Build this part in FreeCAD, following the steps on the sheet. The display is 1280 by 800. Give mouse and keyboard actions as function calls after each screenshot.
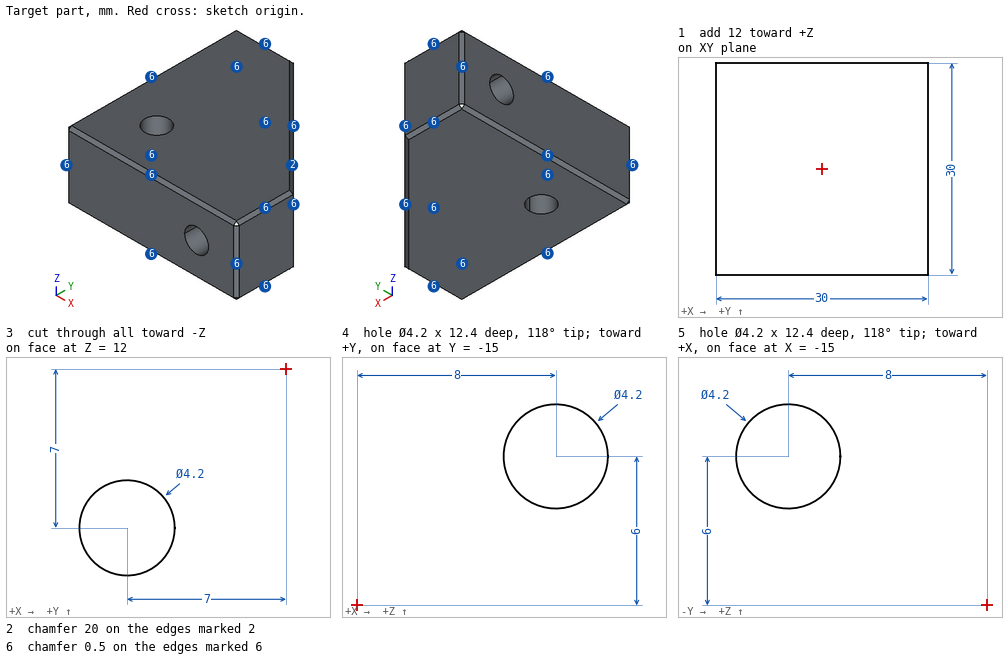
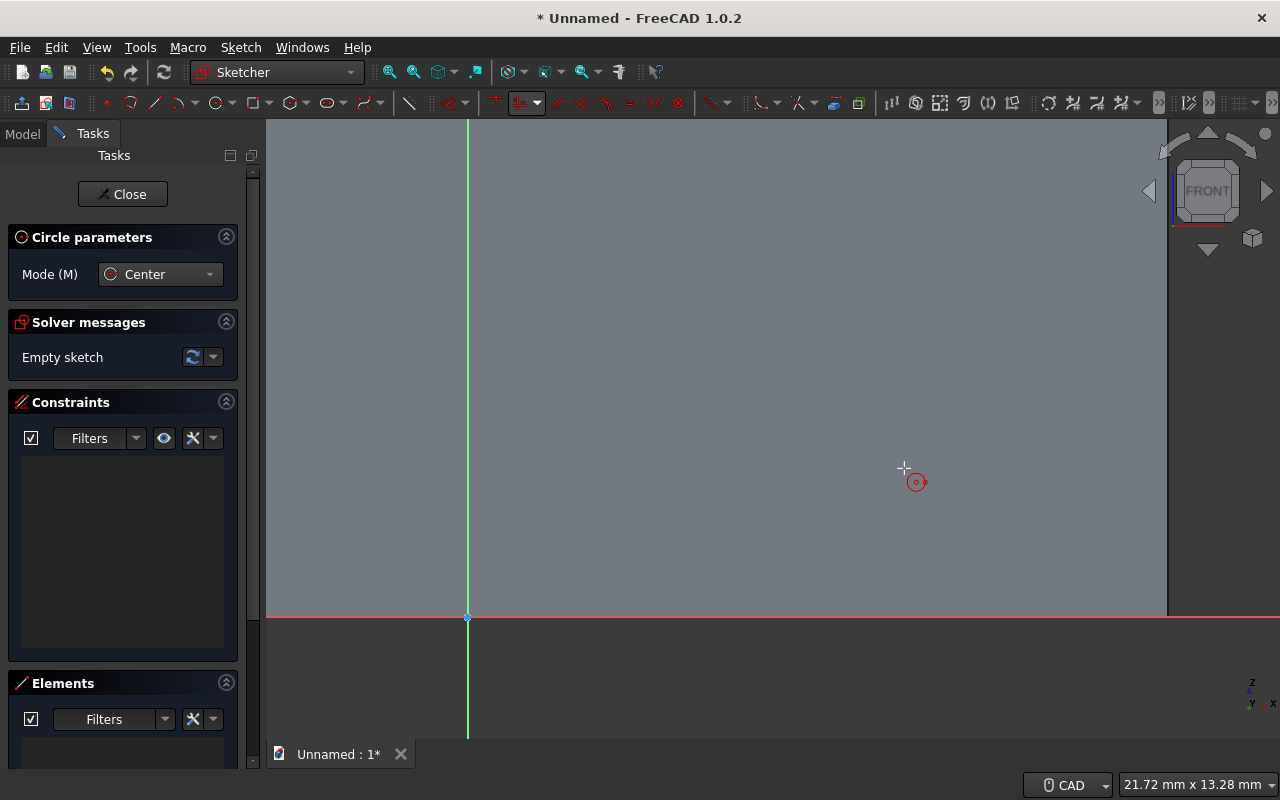
click(841, 337)
click(910, 268)
key(Escape)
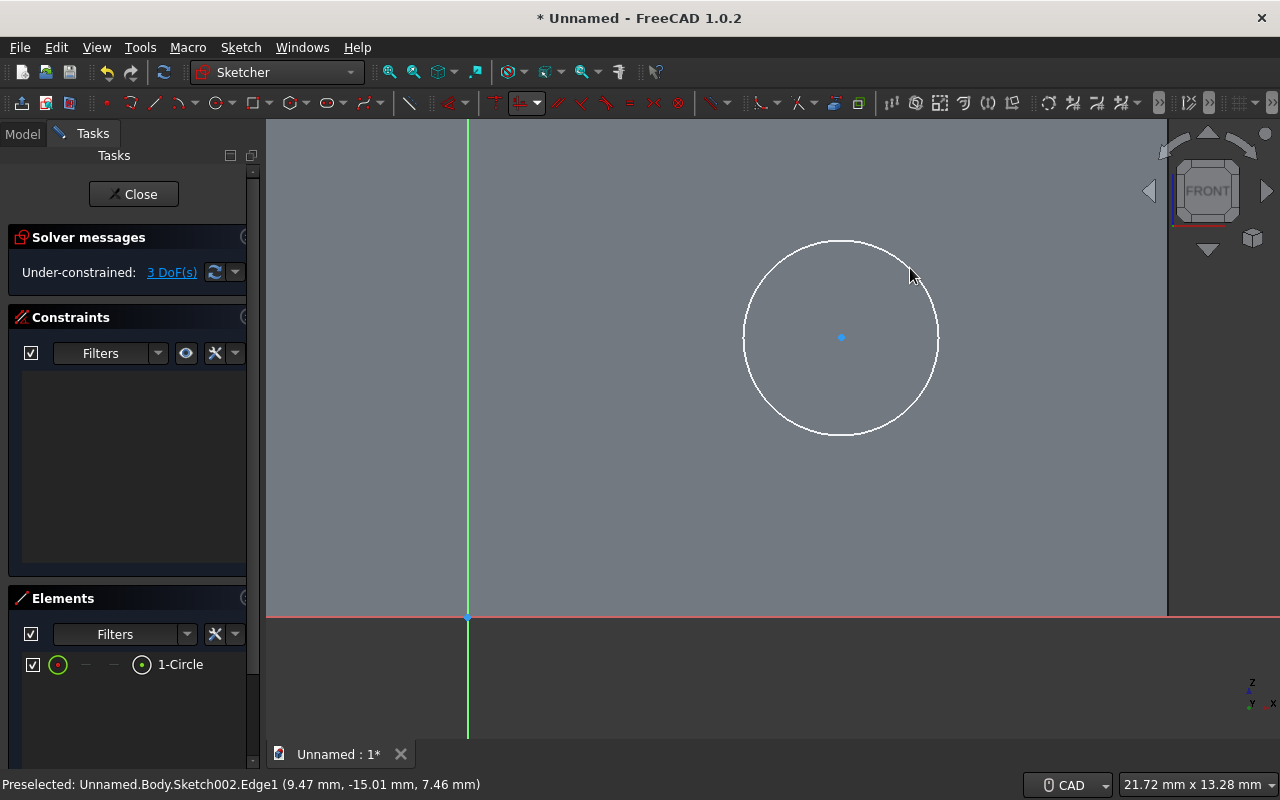
click(448, 104)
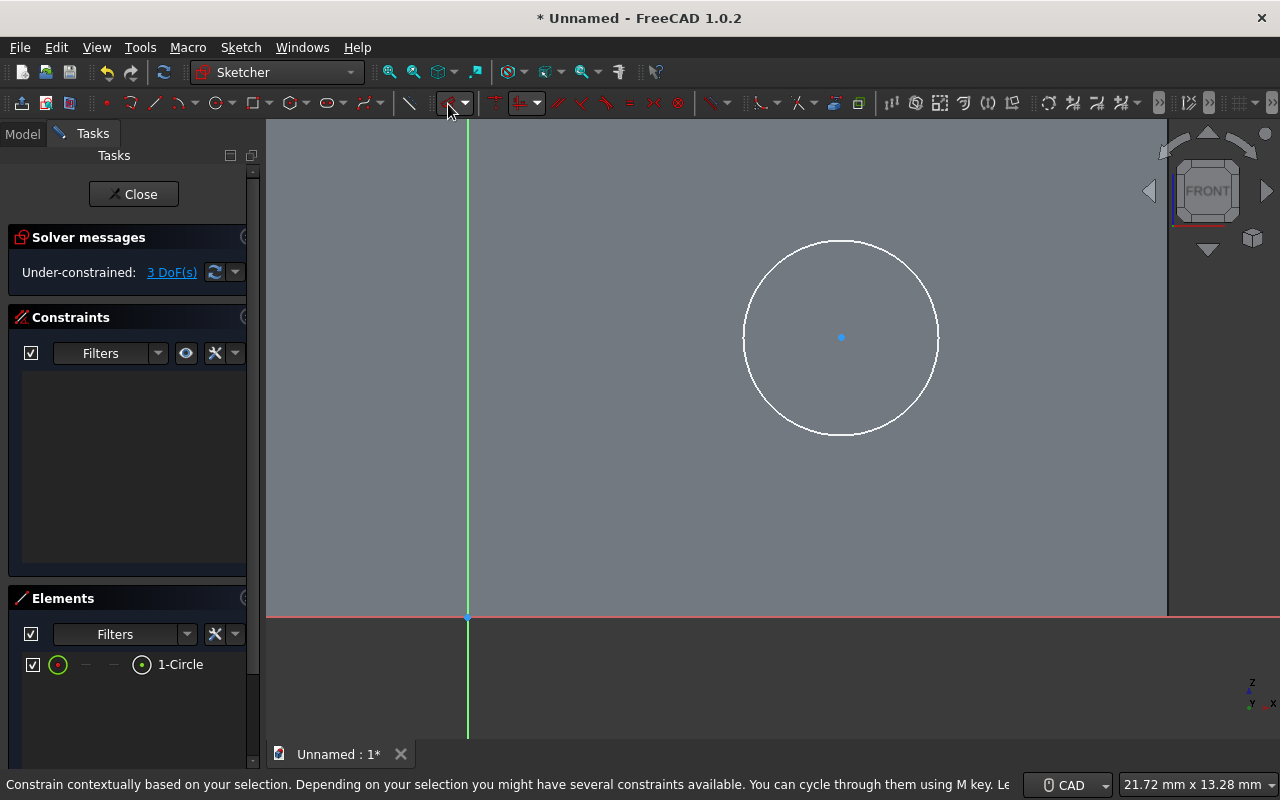
click(910, 269)
click(933, 246)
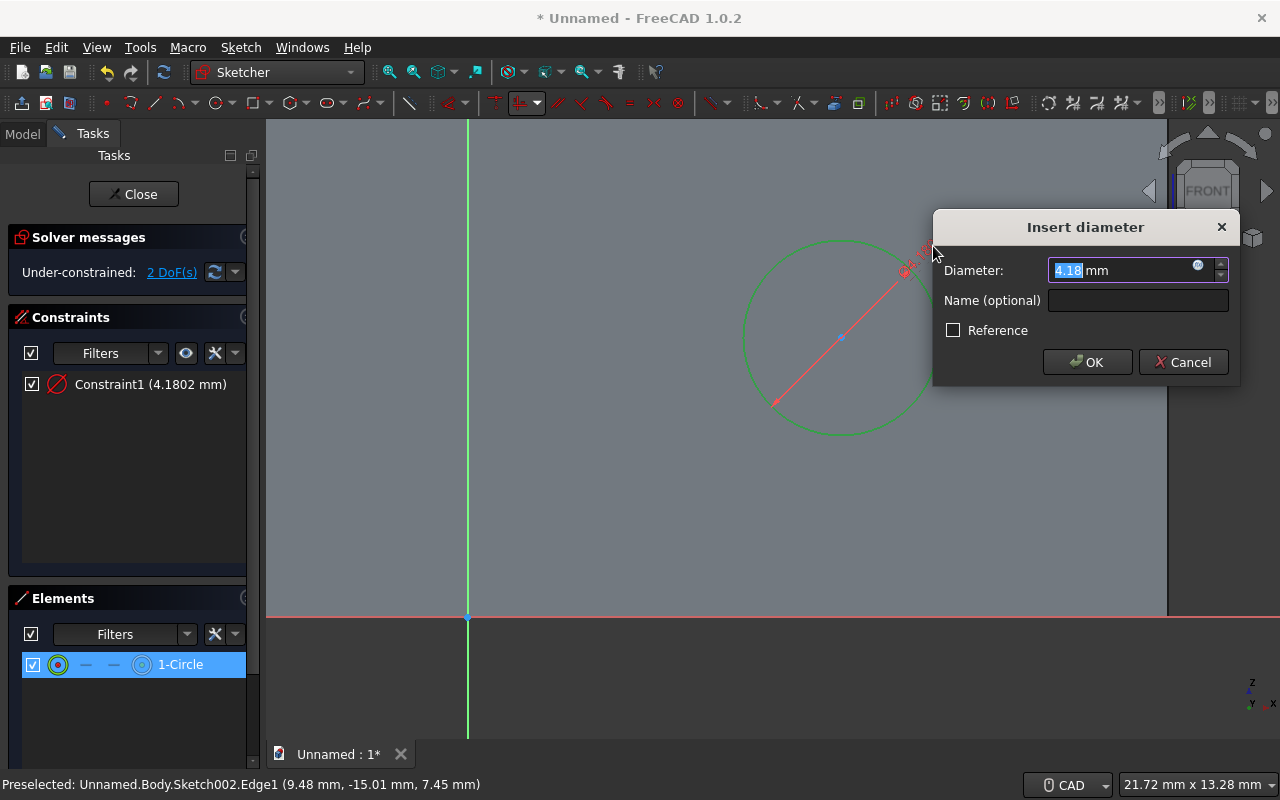
text(4.2)
key(Return)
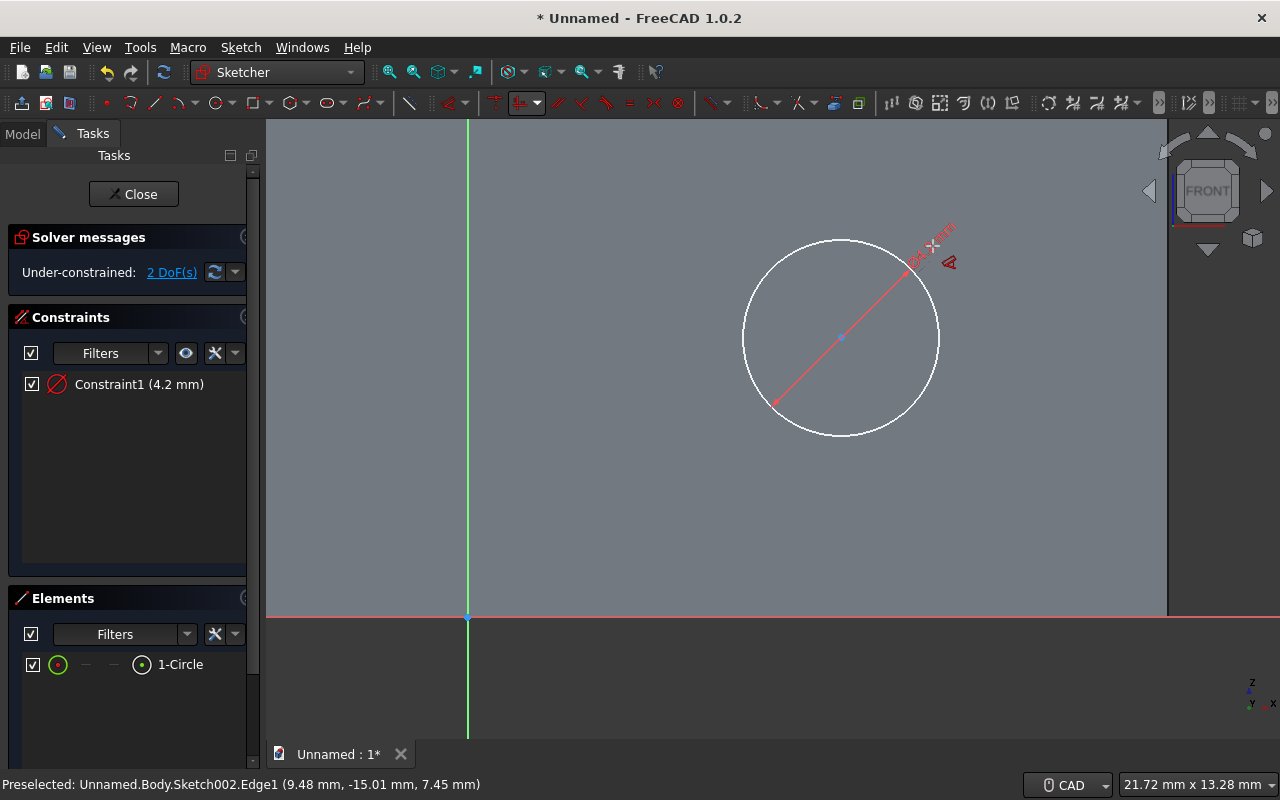
click(841, 338)
click(654, 651)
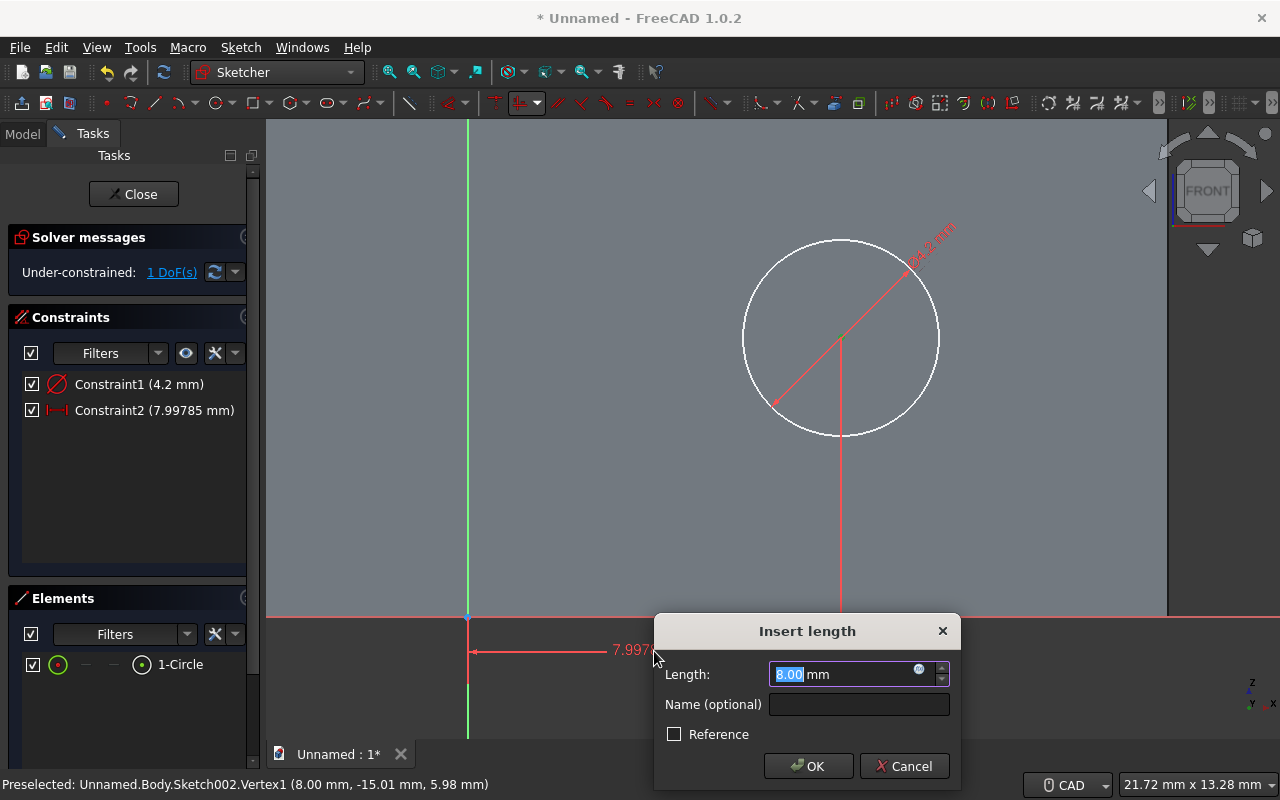
text(8)
key(Return)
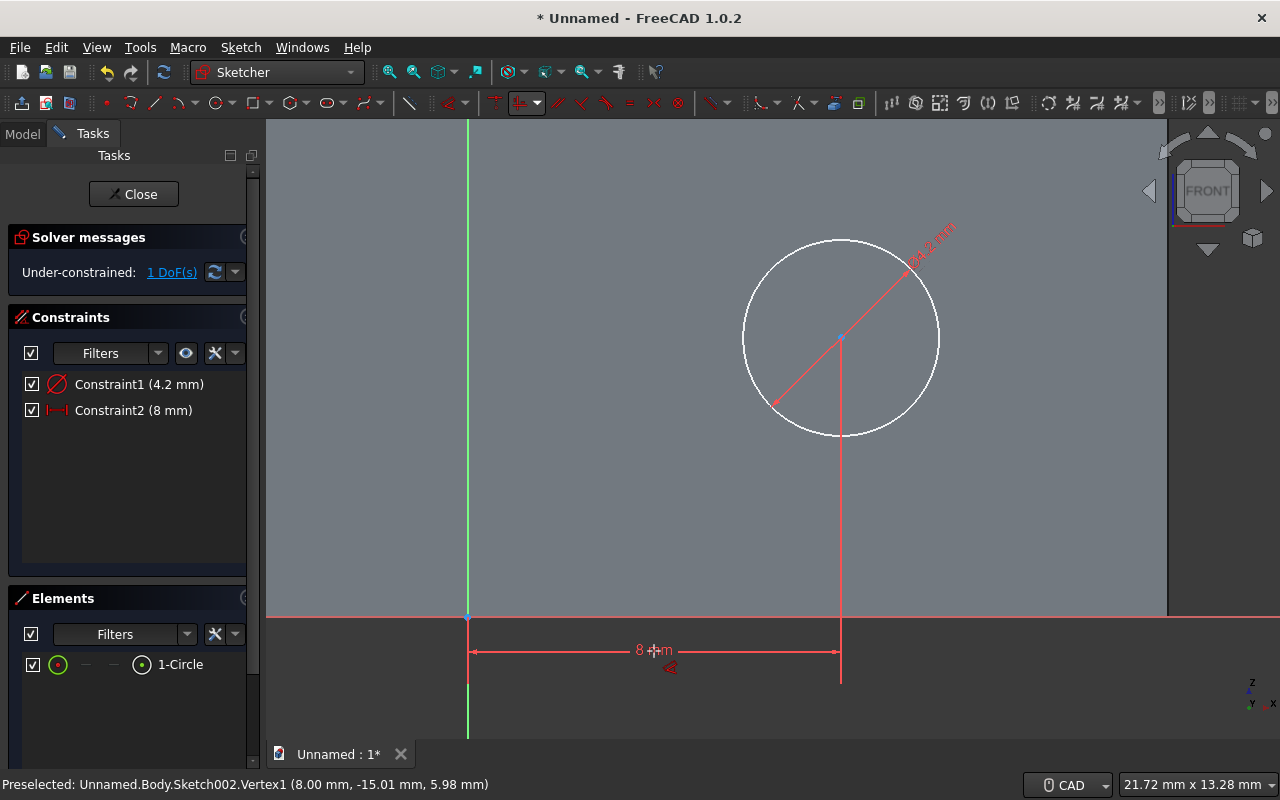
click(841, 338)
click(434, 478)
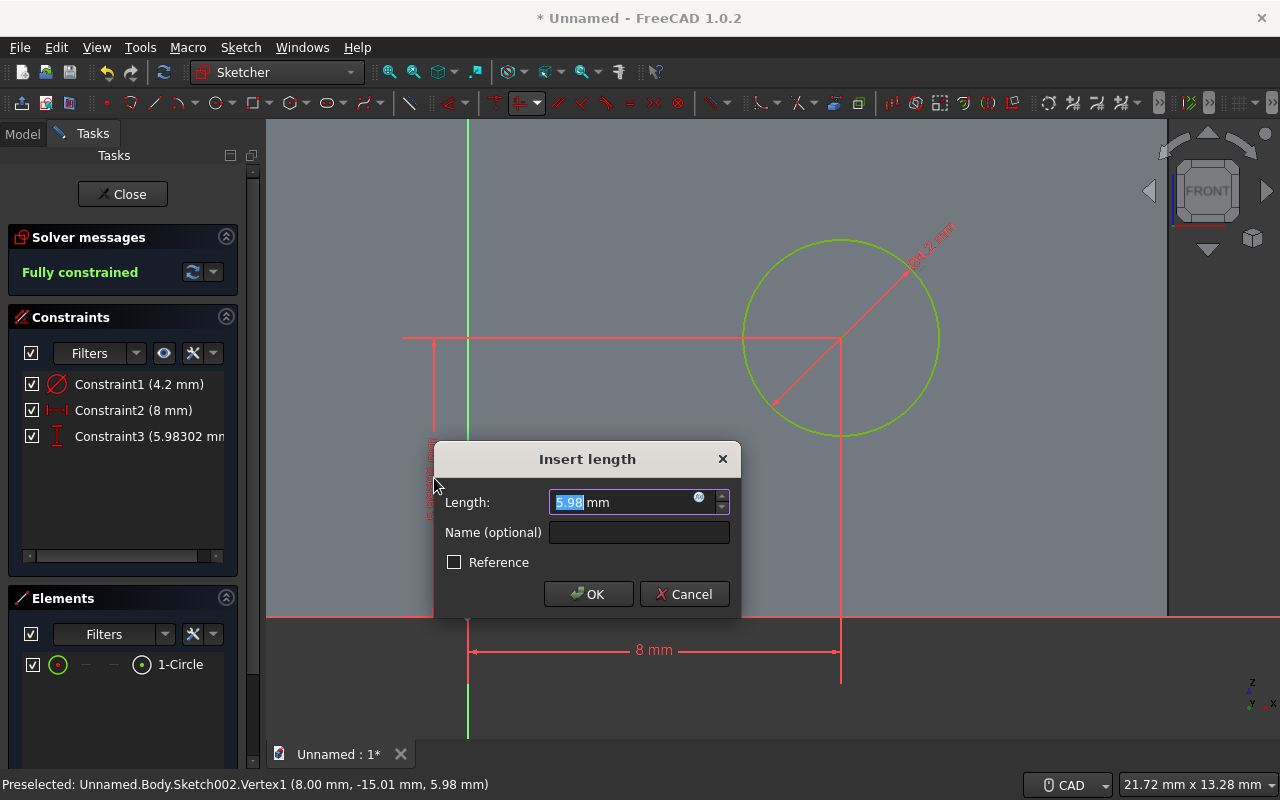
text(6)
key(Return)
key(Escape)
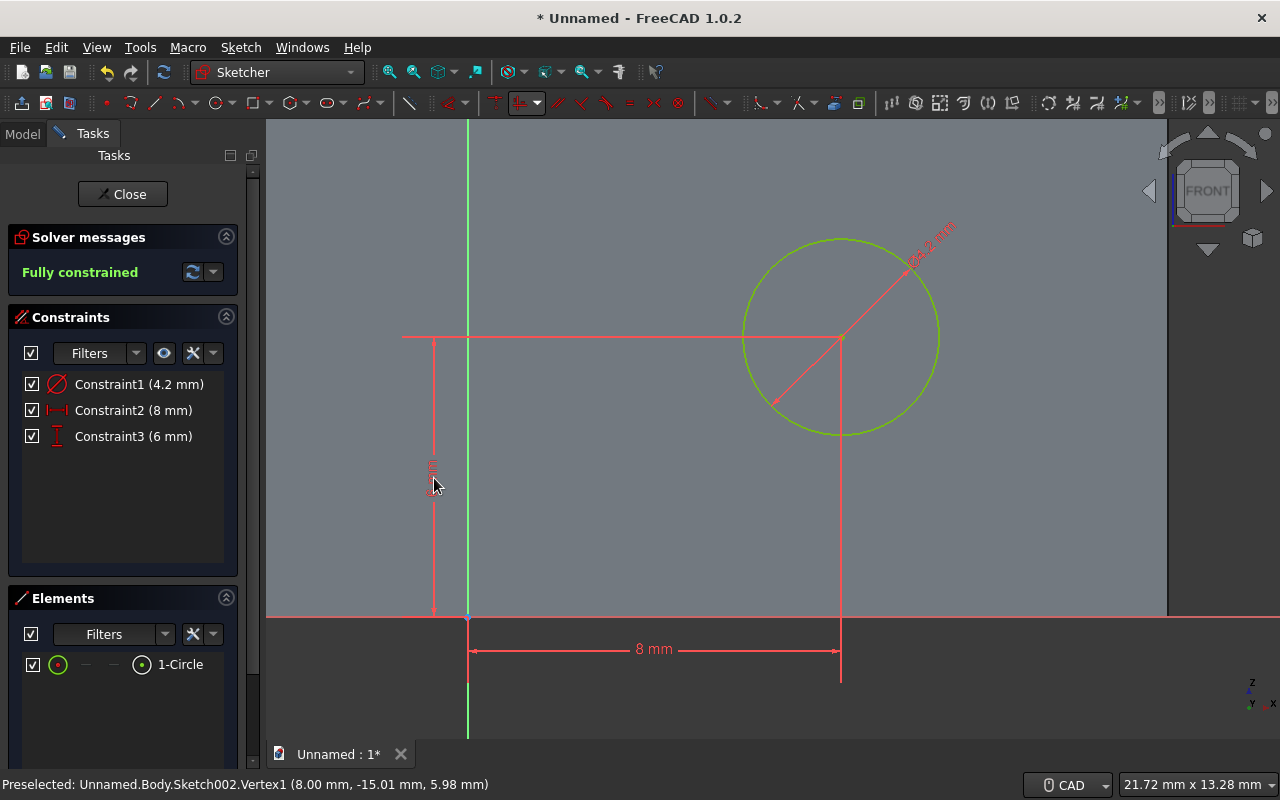
click(123, 194)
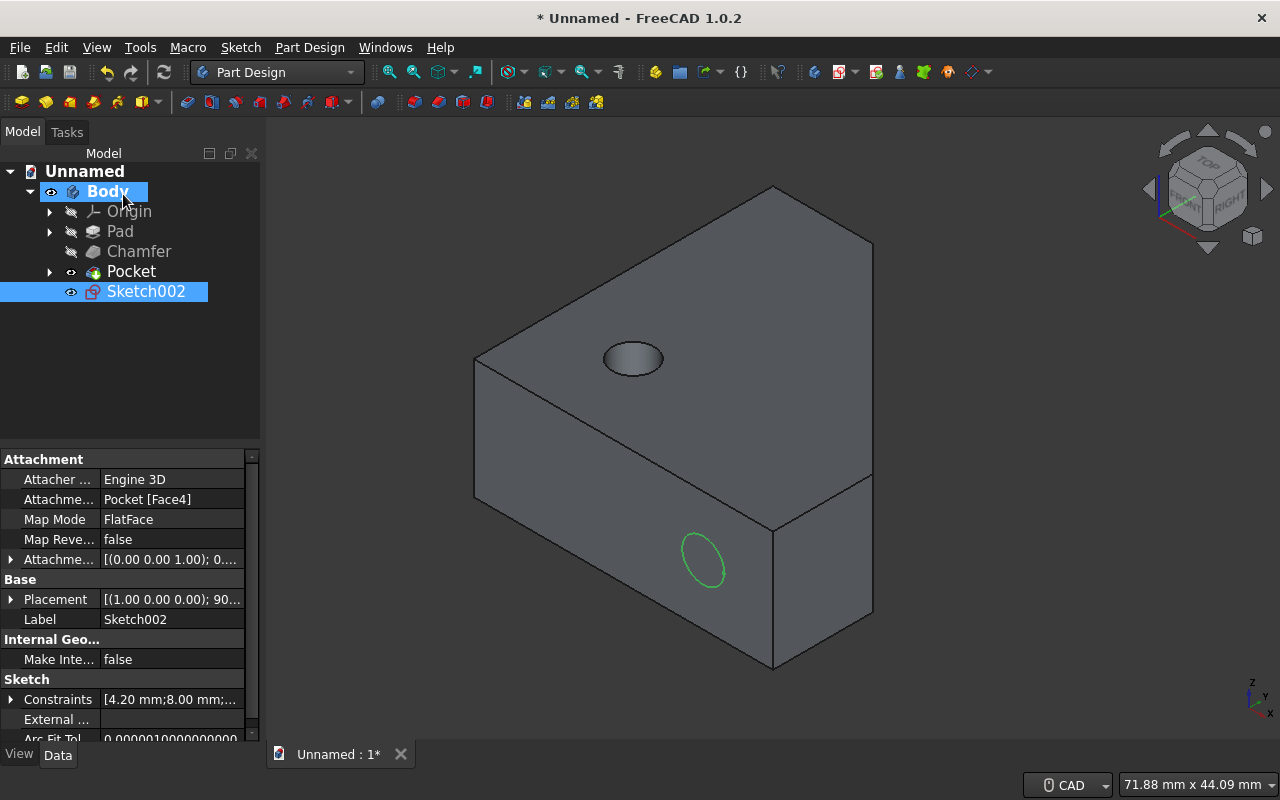
click(212, 102)